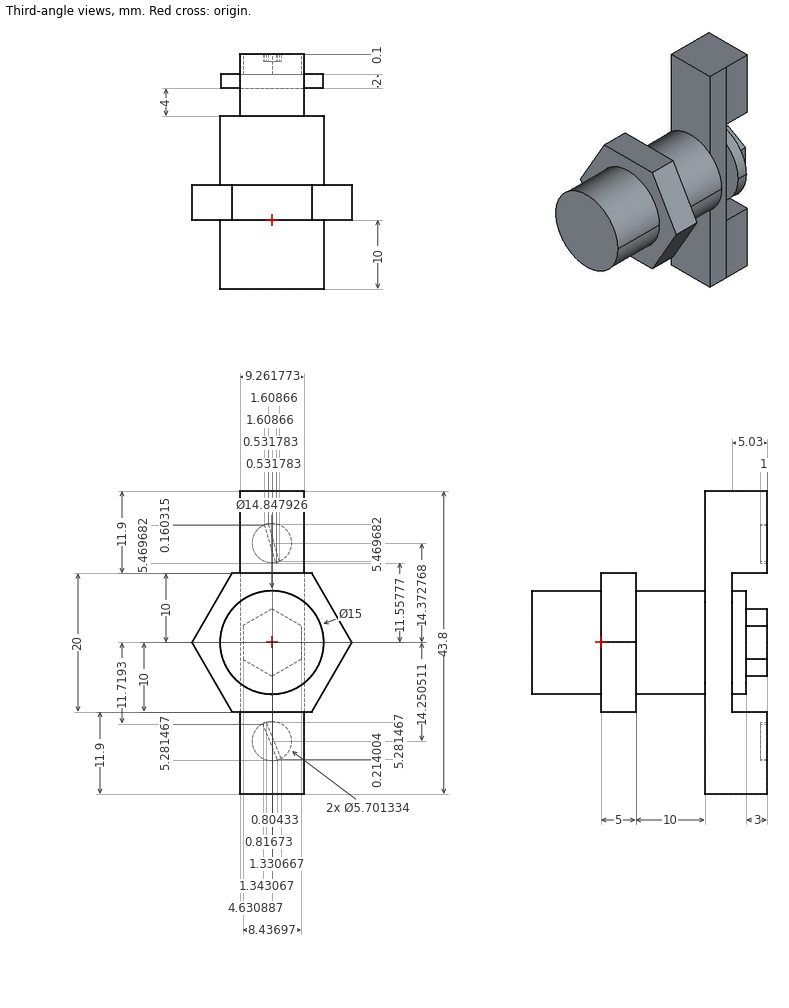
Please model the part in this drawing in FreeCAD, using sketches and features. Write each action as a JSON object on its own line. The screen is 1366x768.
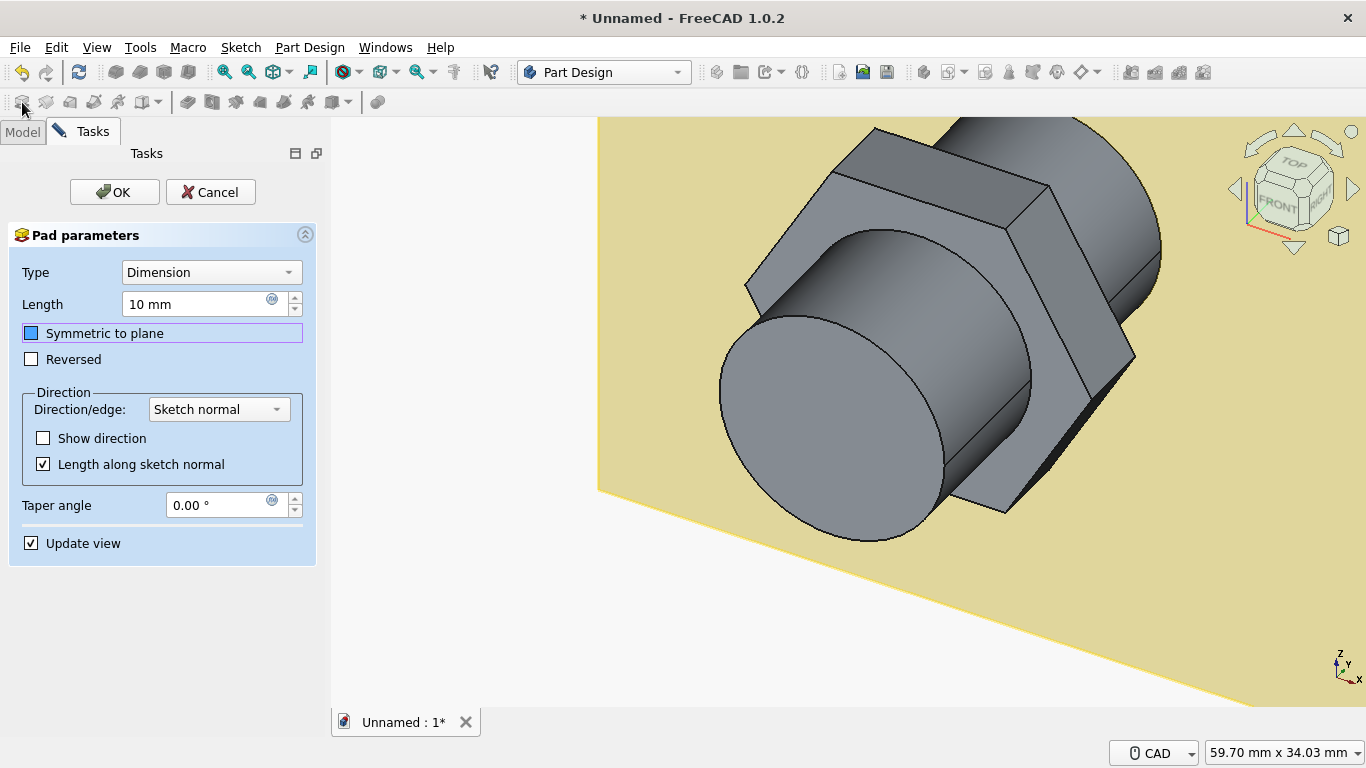
{"action": "left_click", "coordinate": [115, 192]}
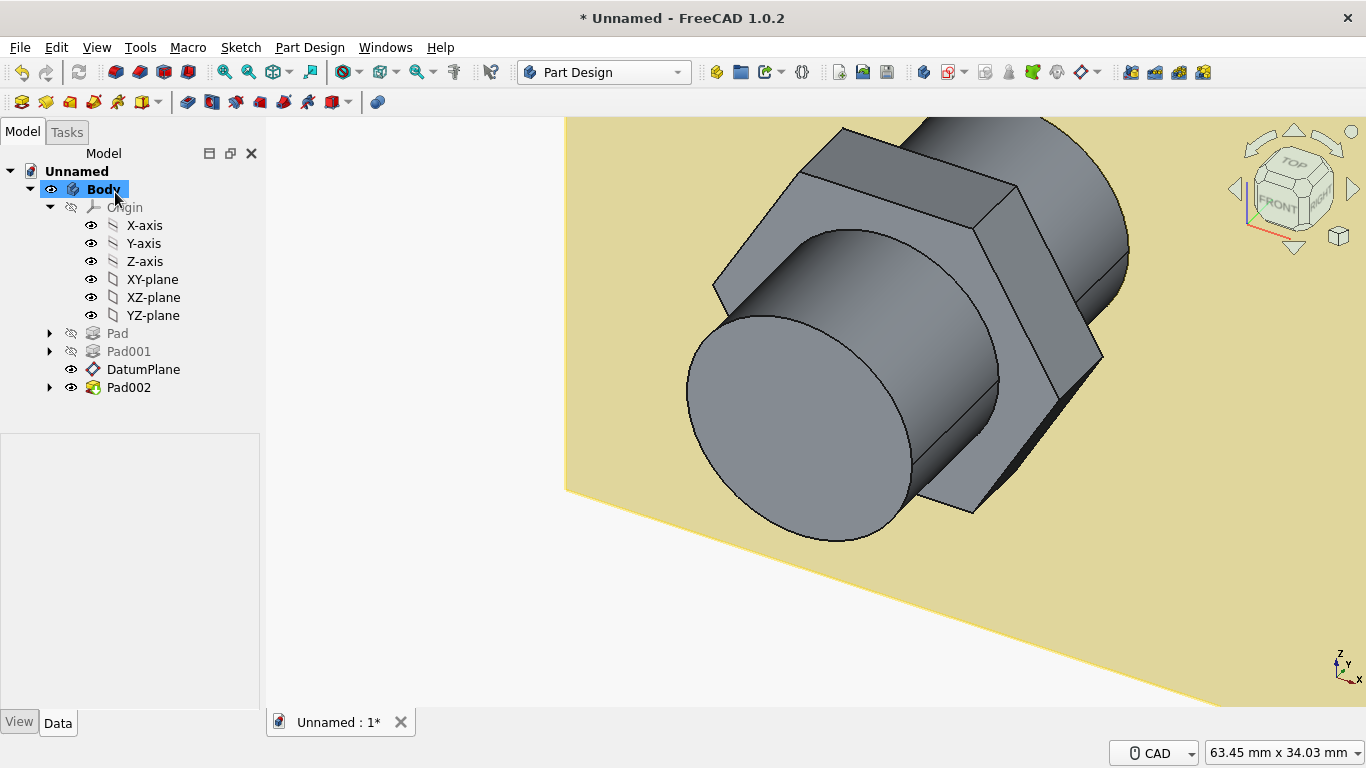
{"action": "left_click", "coordinate": [116, 369]}
{"action": "key", "text": "space"}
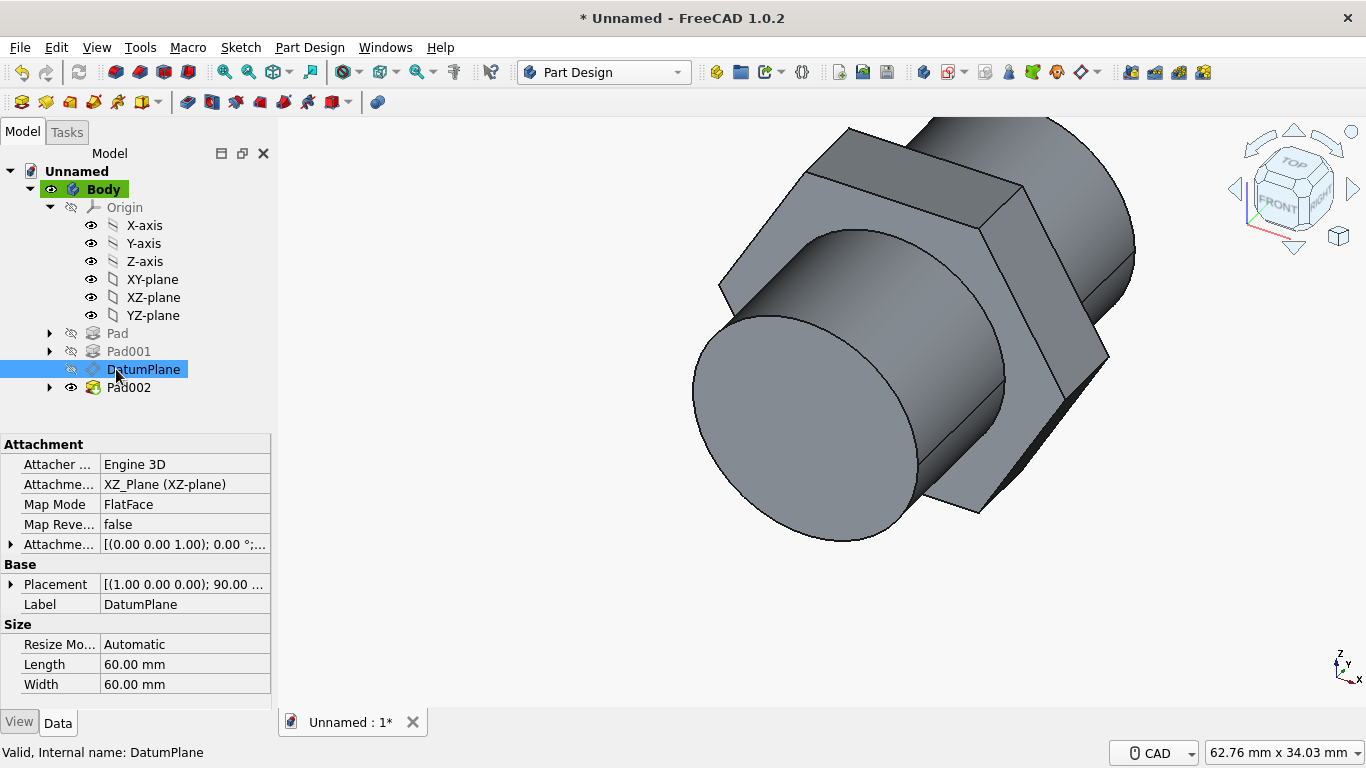
{"action": "left_click", "coordinate": [226, 72]}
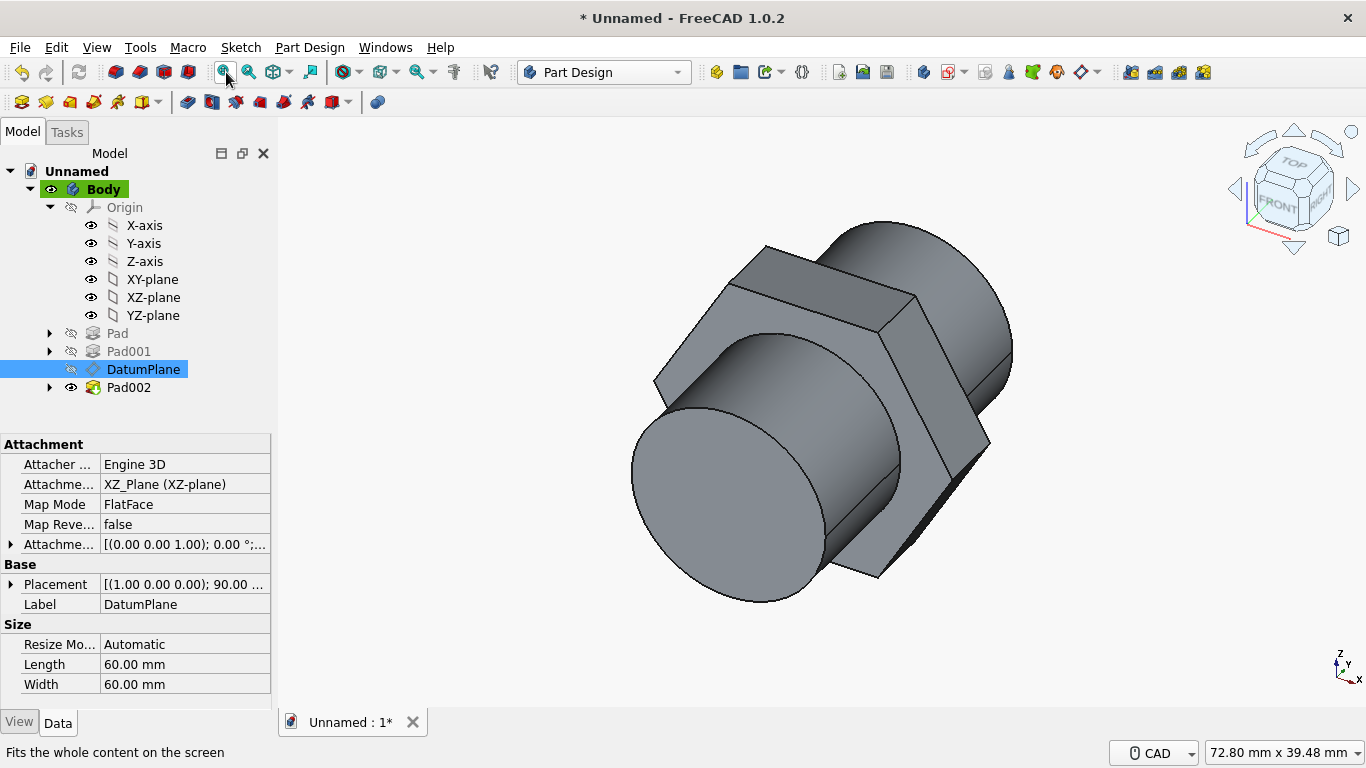
{"action": "key", "text": "4"}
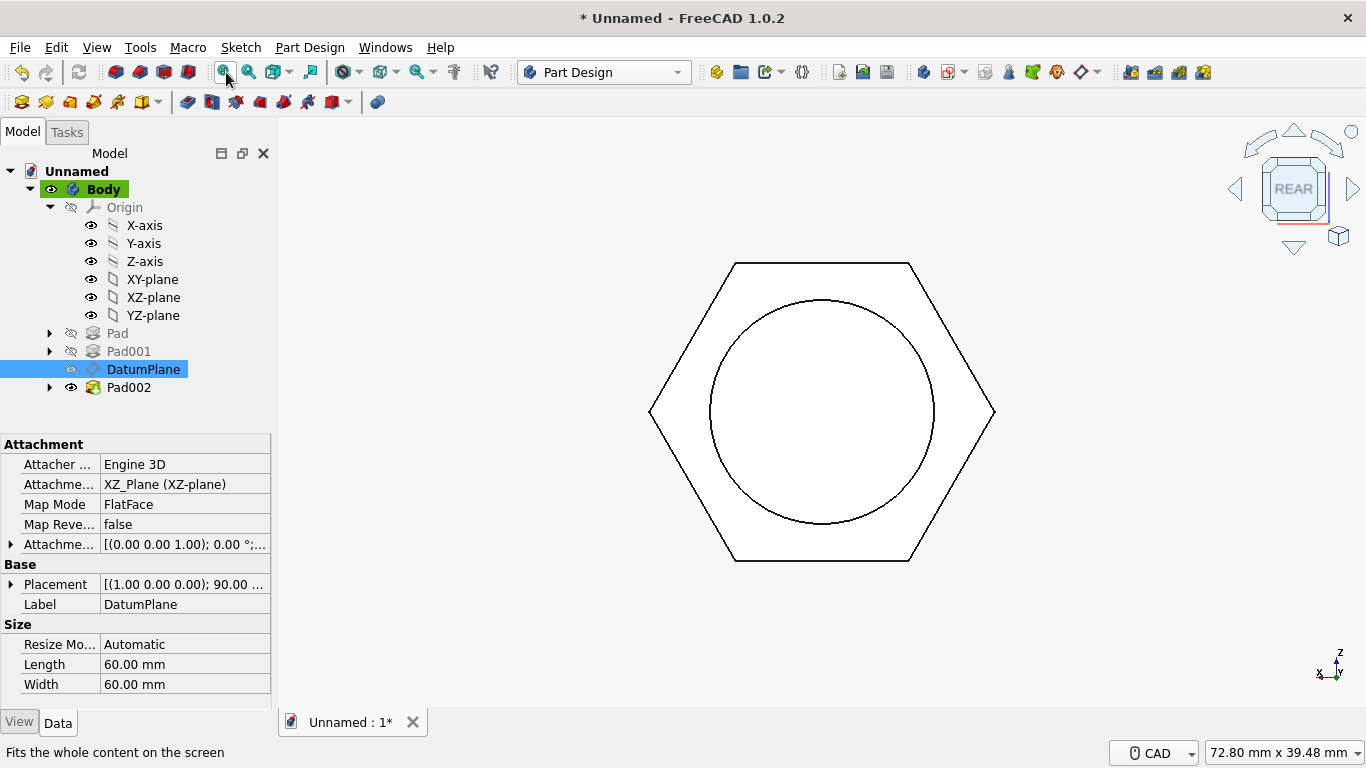
{"action": "left_click", "coordinate": [822, 411]}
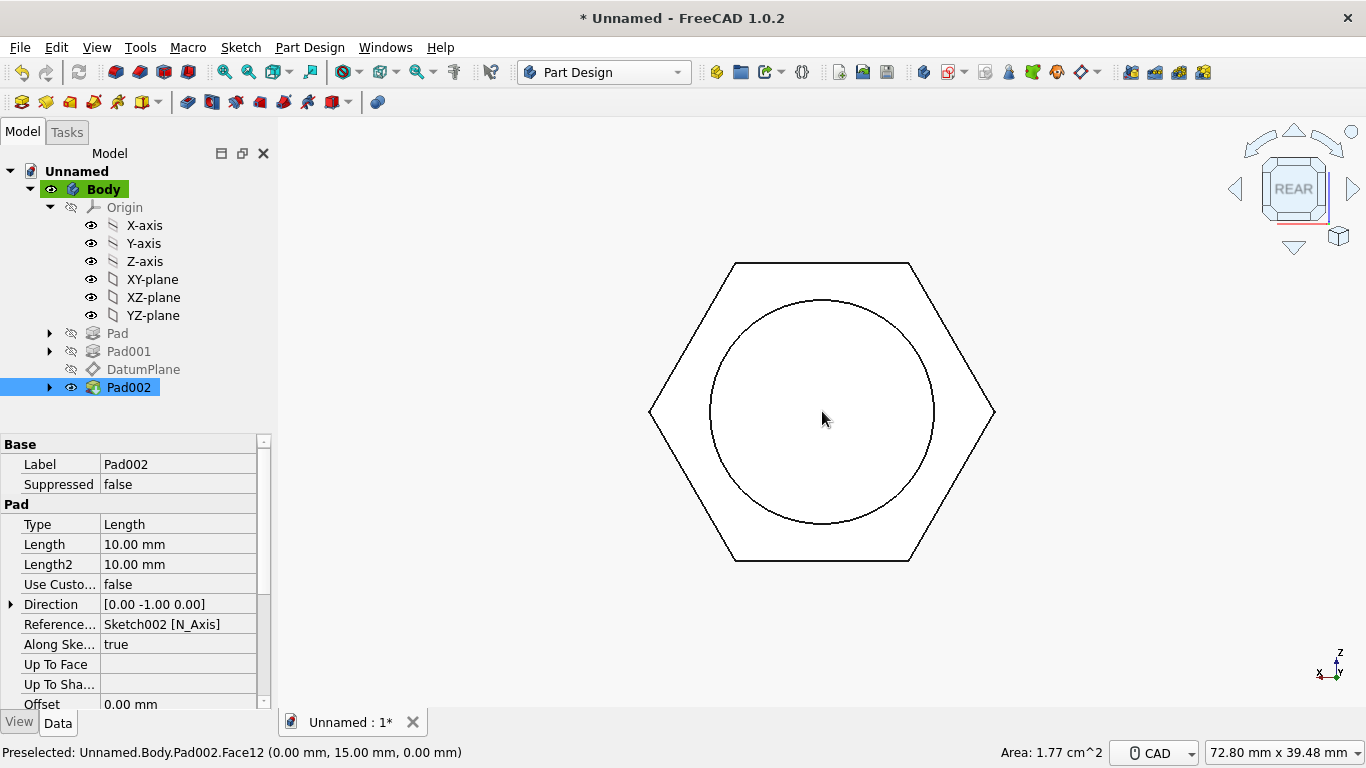
{"action": "left_click", "coordinate": [948, 72]}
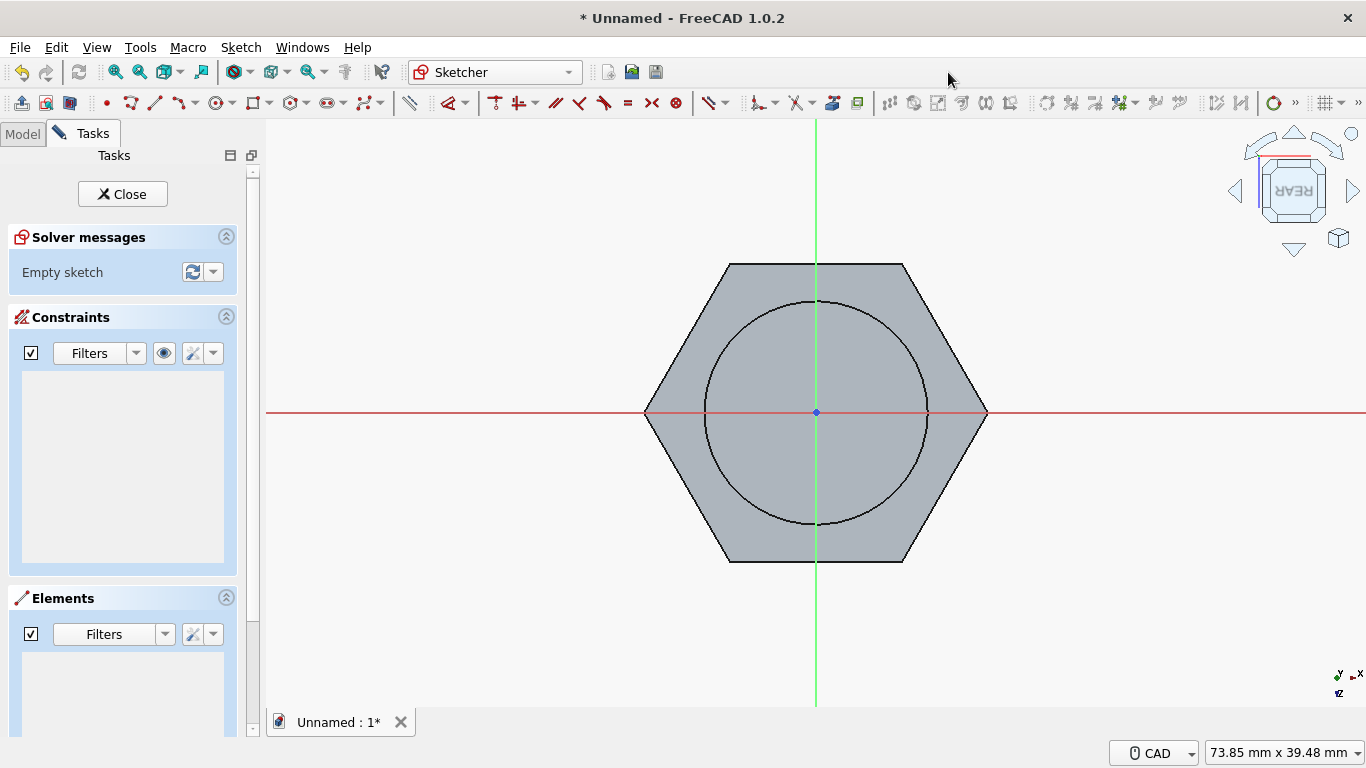
{"action": "scroll", "coordinate": [664, 413], "scroll_direction": "down", "scroll_amount": 3}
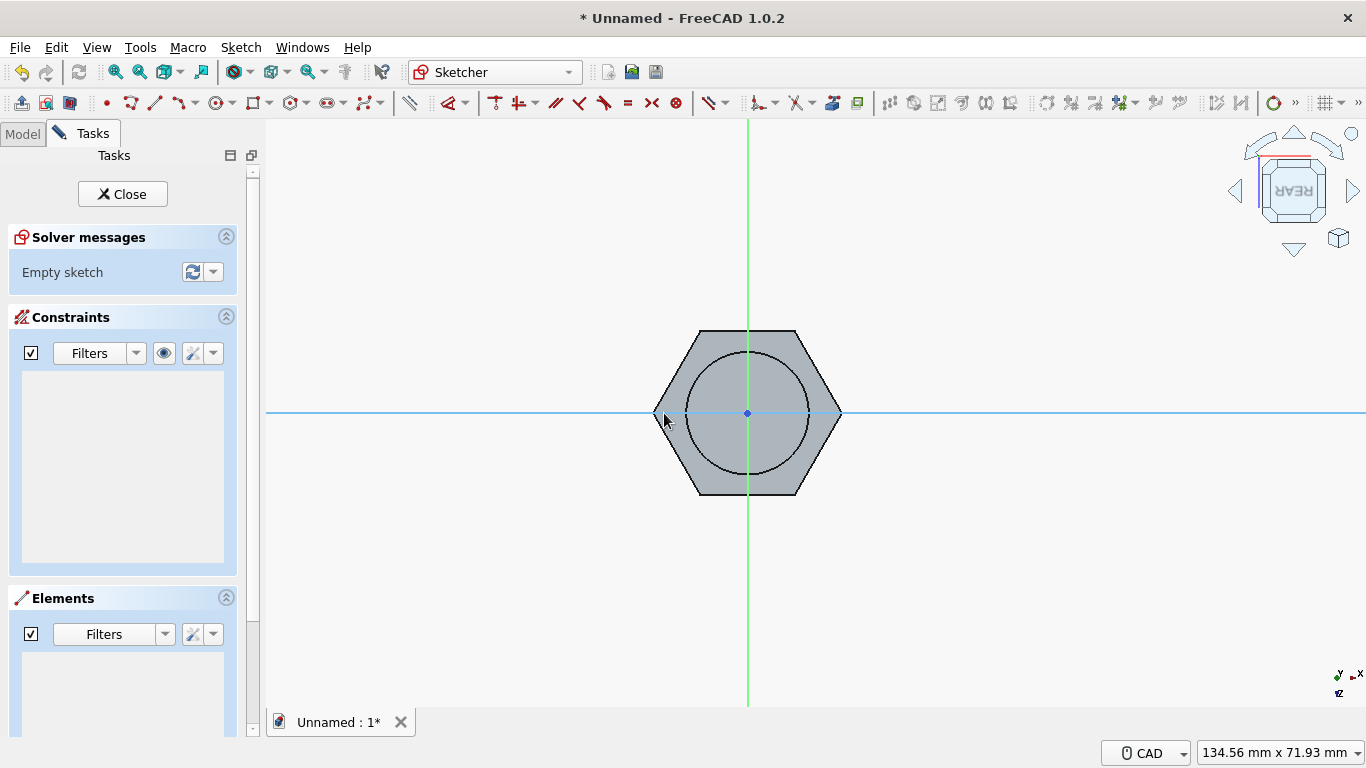
{"action": "key", "text": "g v"}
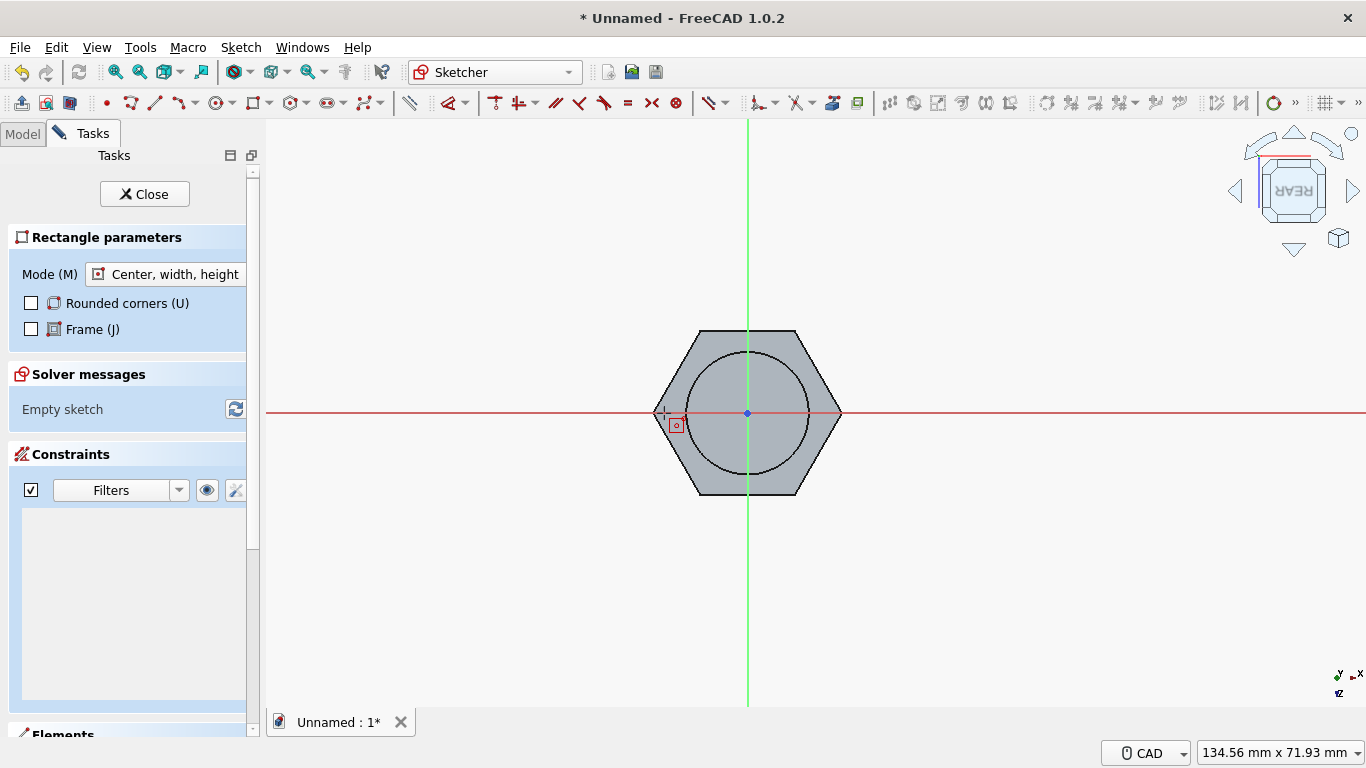
{"action": "left_click", "coordinate": [748, 413]}
{"action": "left_click", "coordinate": [785, 234]}
{"action": "key", "text": "Escape"}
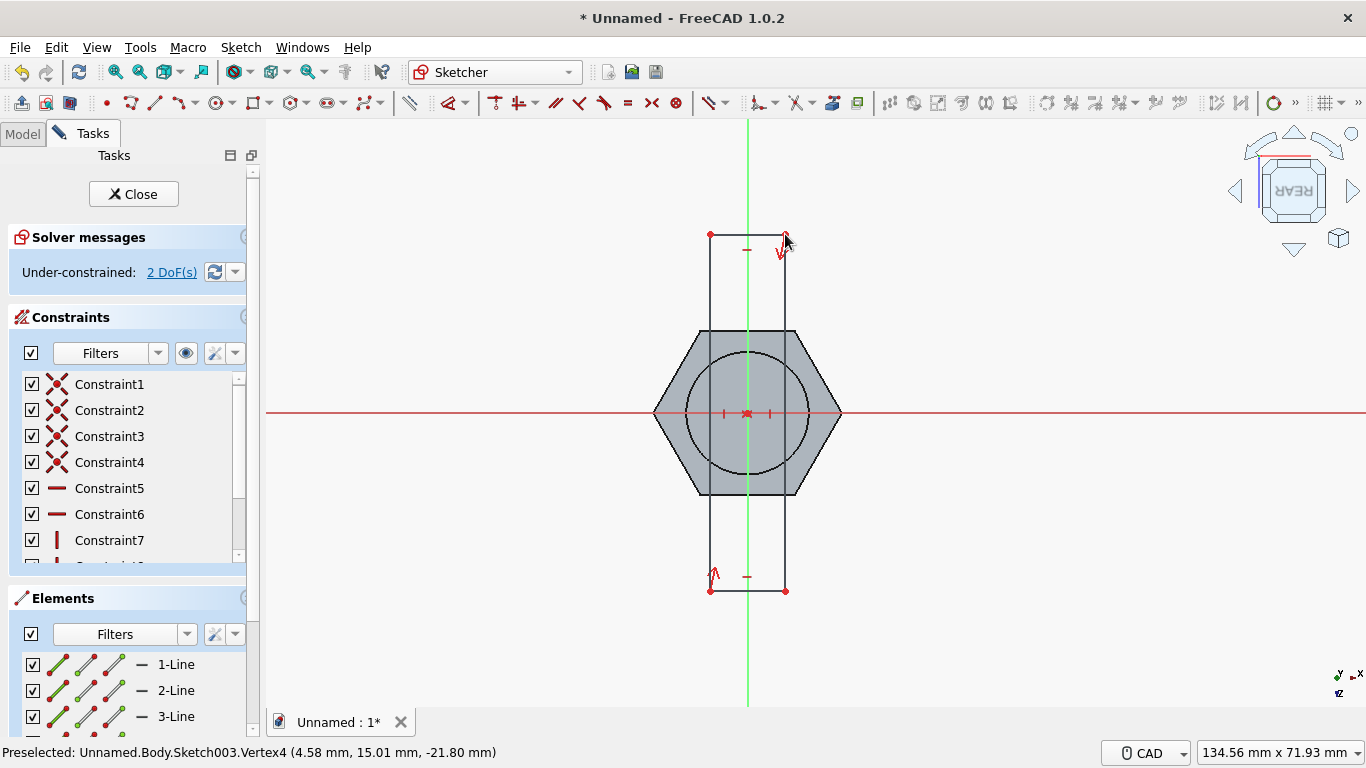
{"action": "left_click", "coordinate": [448, 104]}